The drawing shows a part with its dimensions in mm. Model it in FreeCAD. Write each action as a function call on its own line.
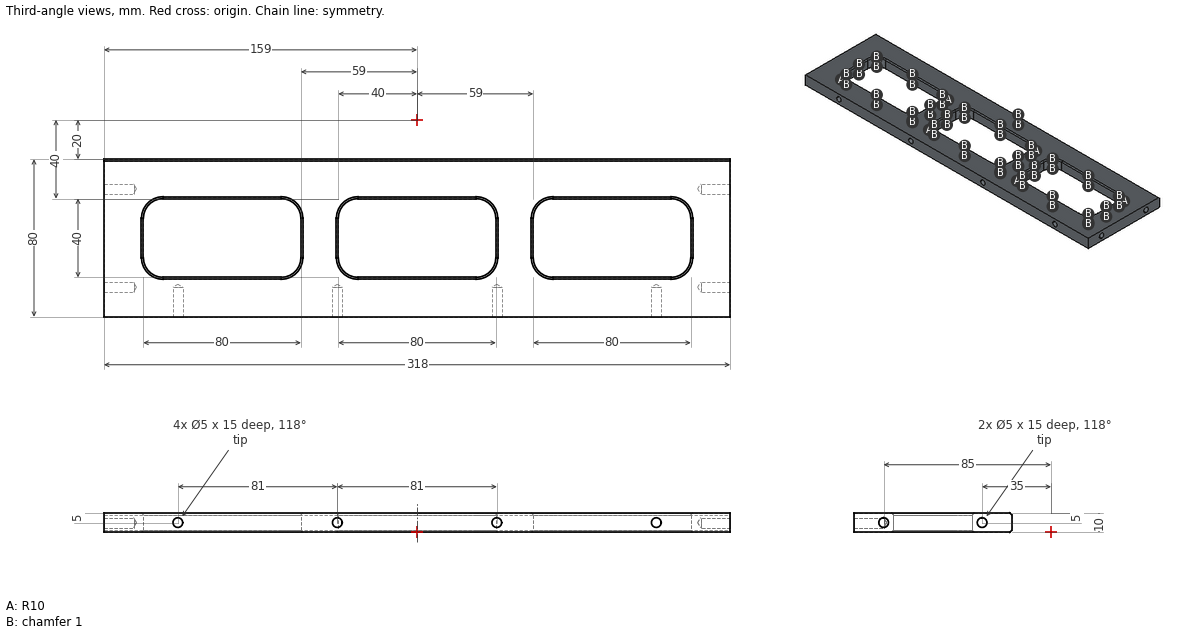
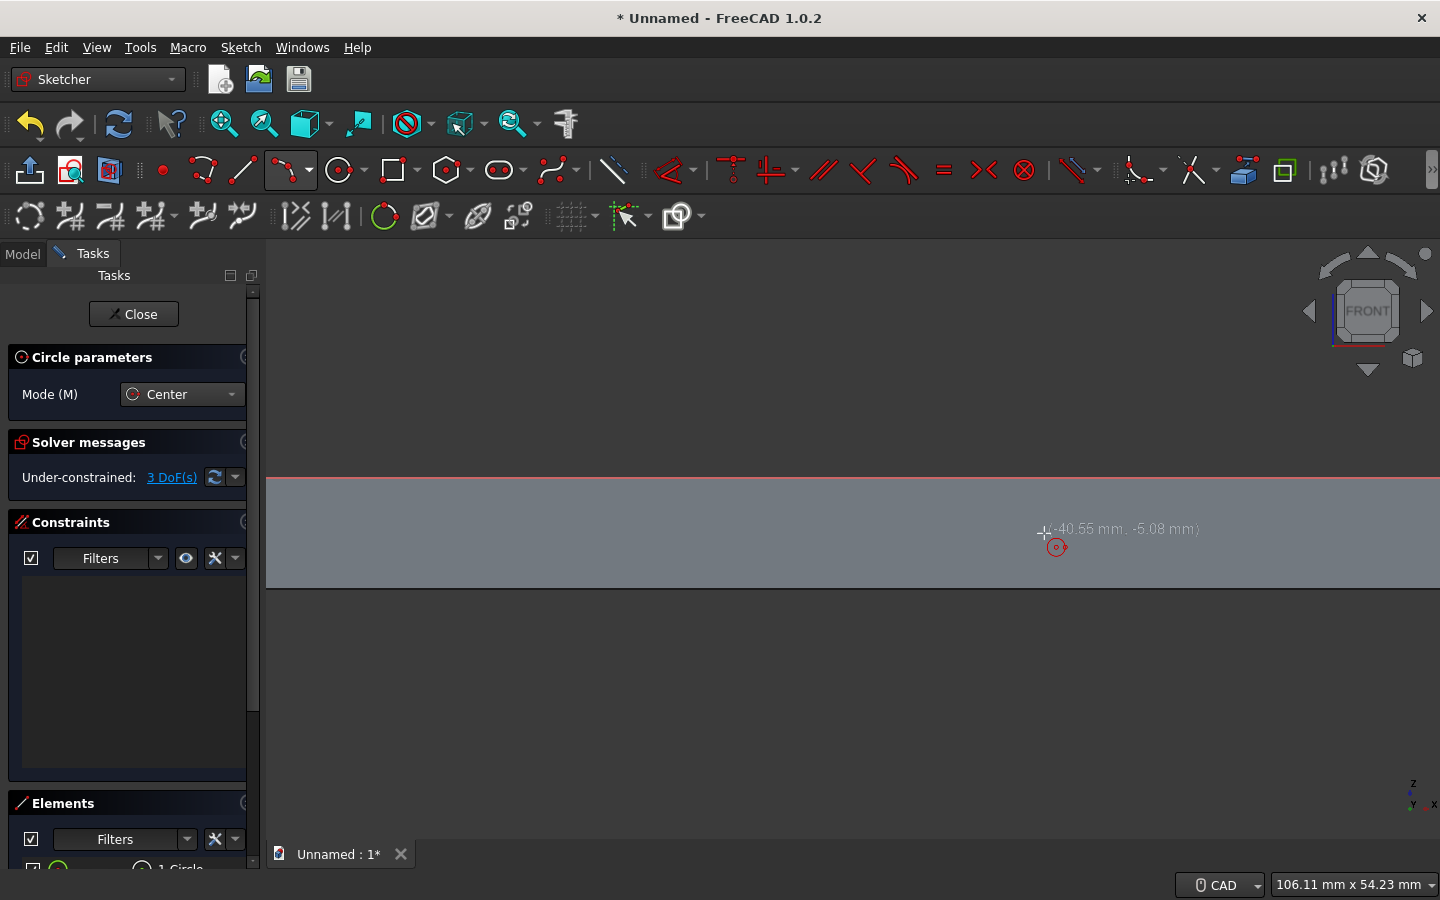
scroll(553, 545, down, 7)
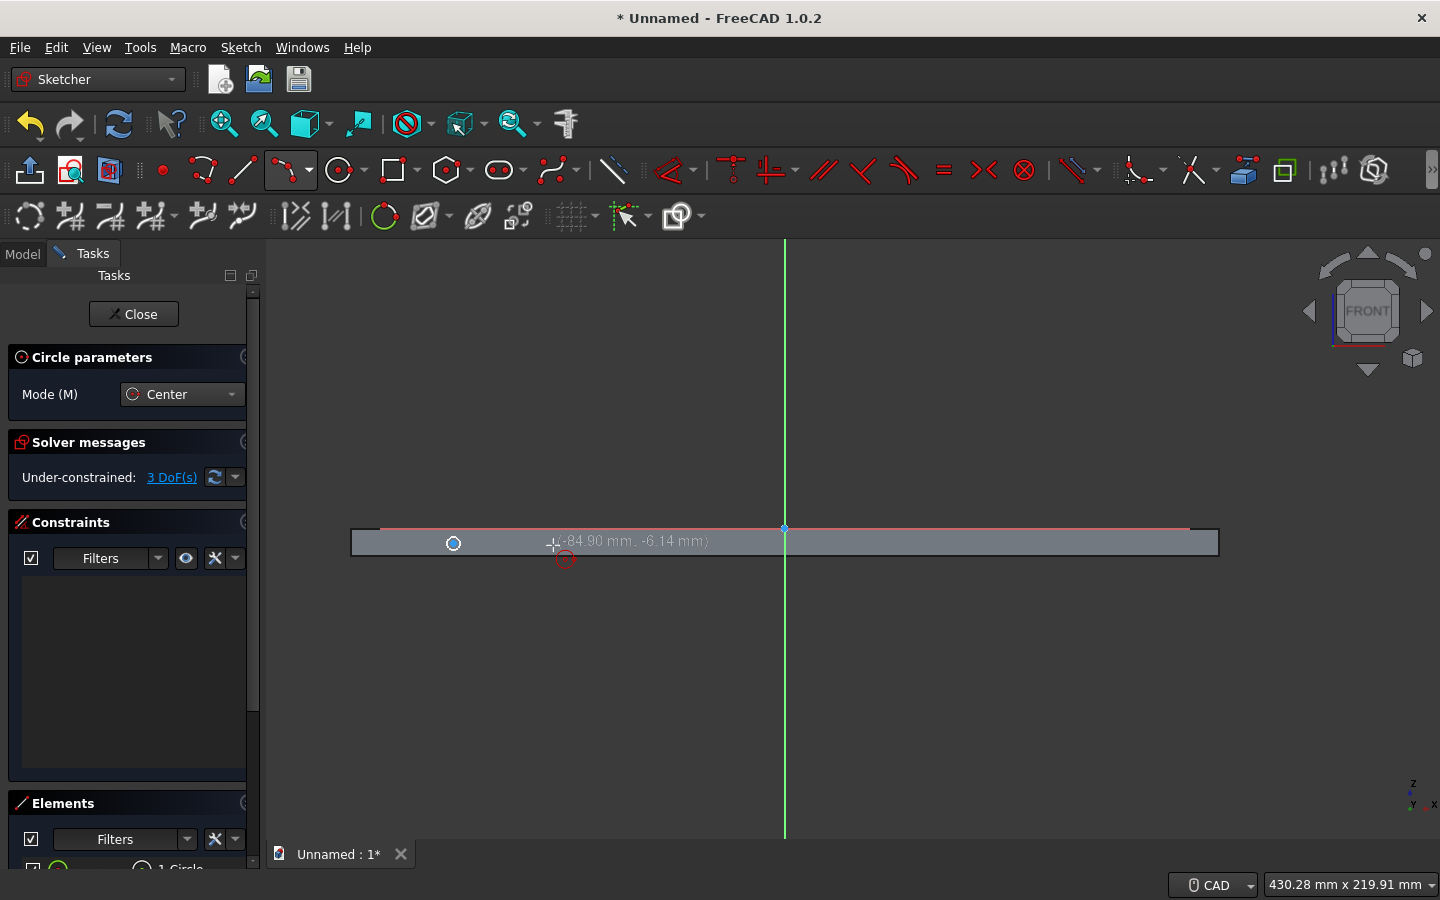
click(674, 543)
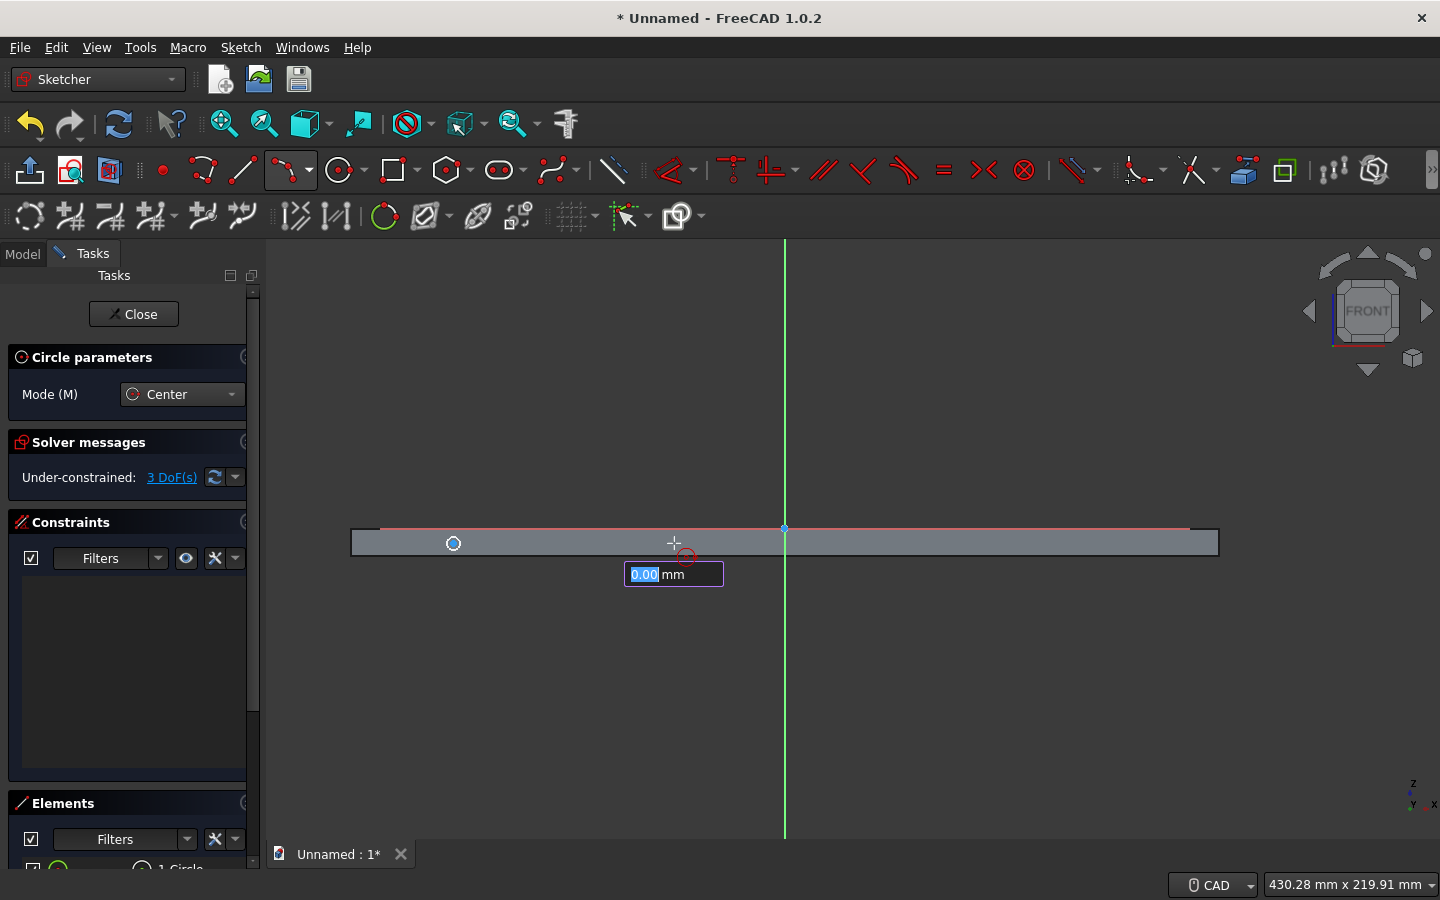
scroll(679, 547, up, 5)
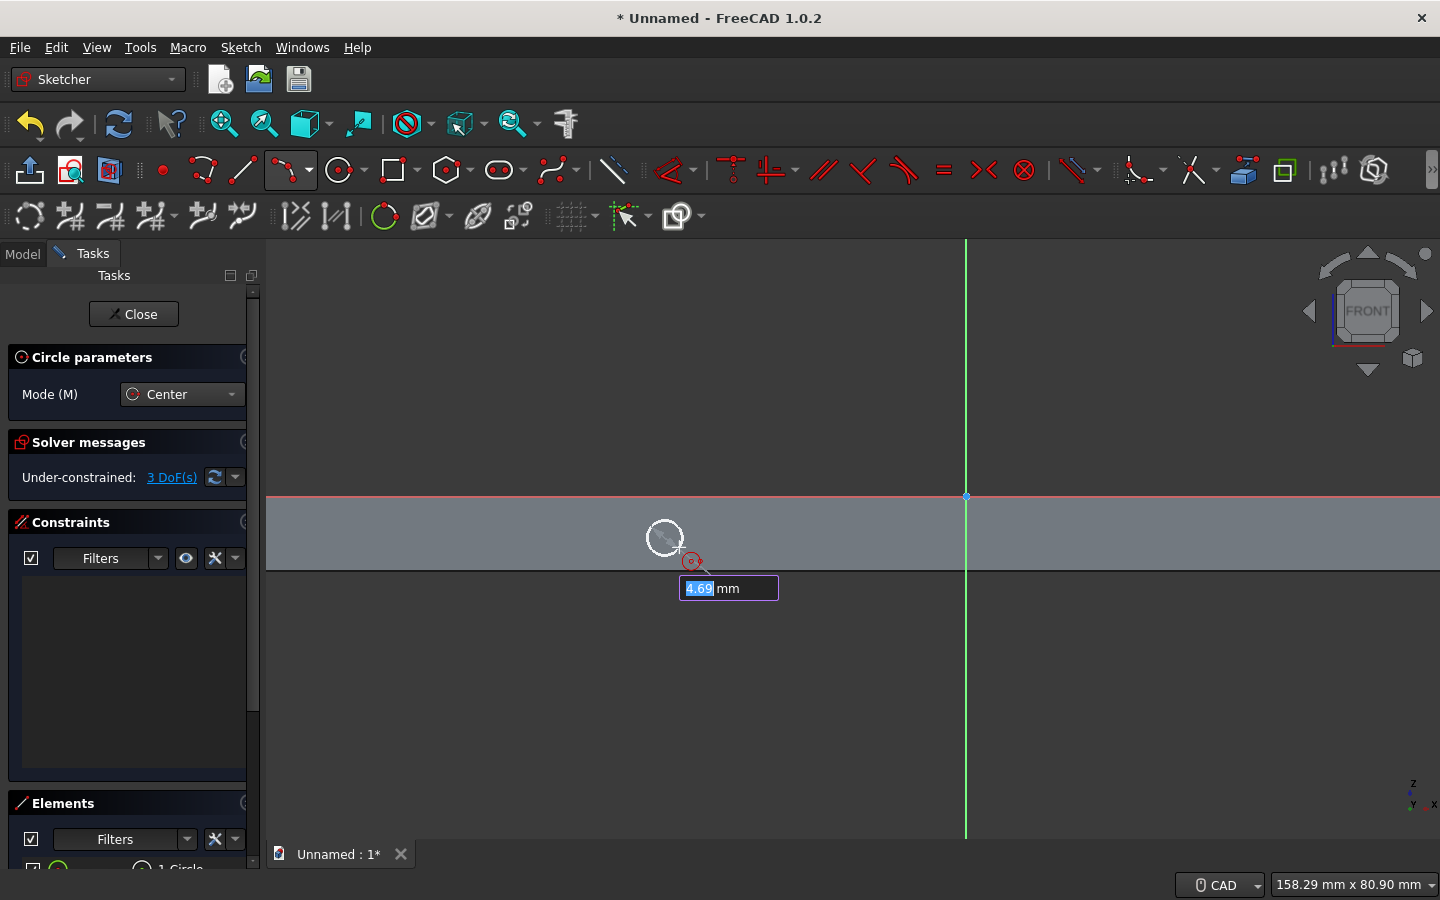
click(679, 547)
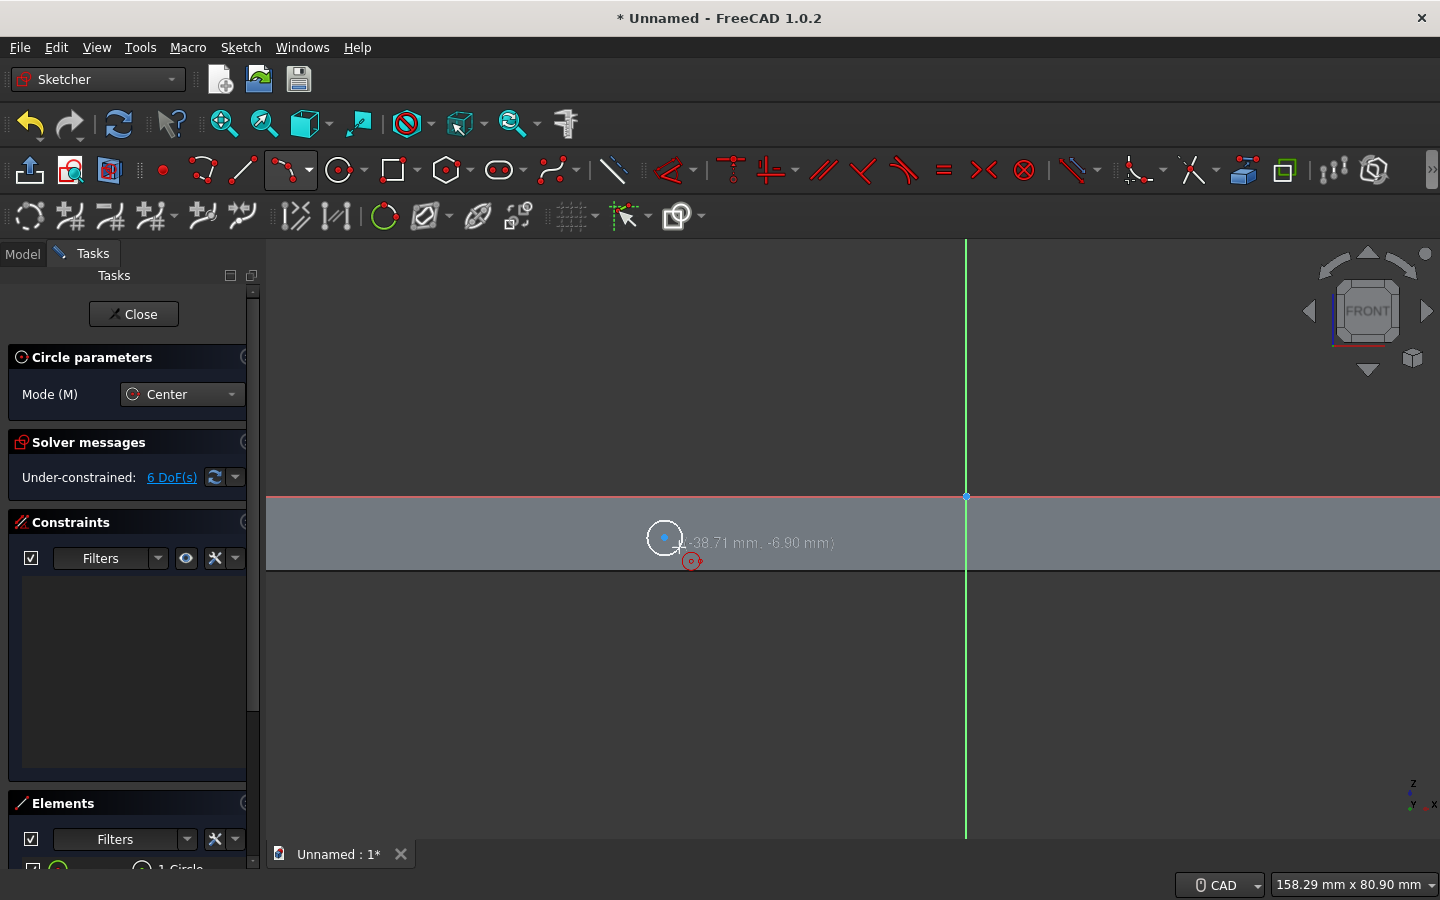
scroll(1266, 534, up, 2)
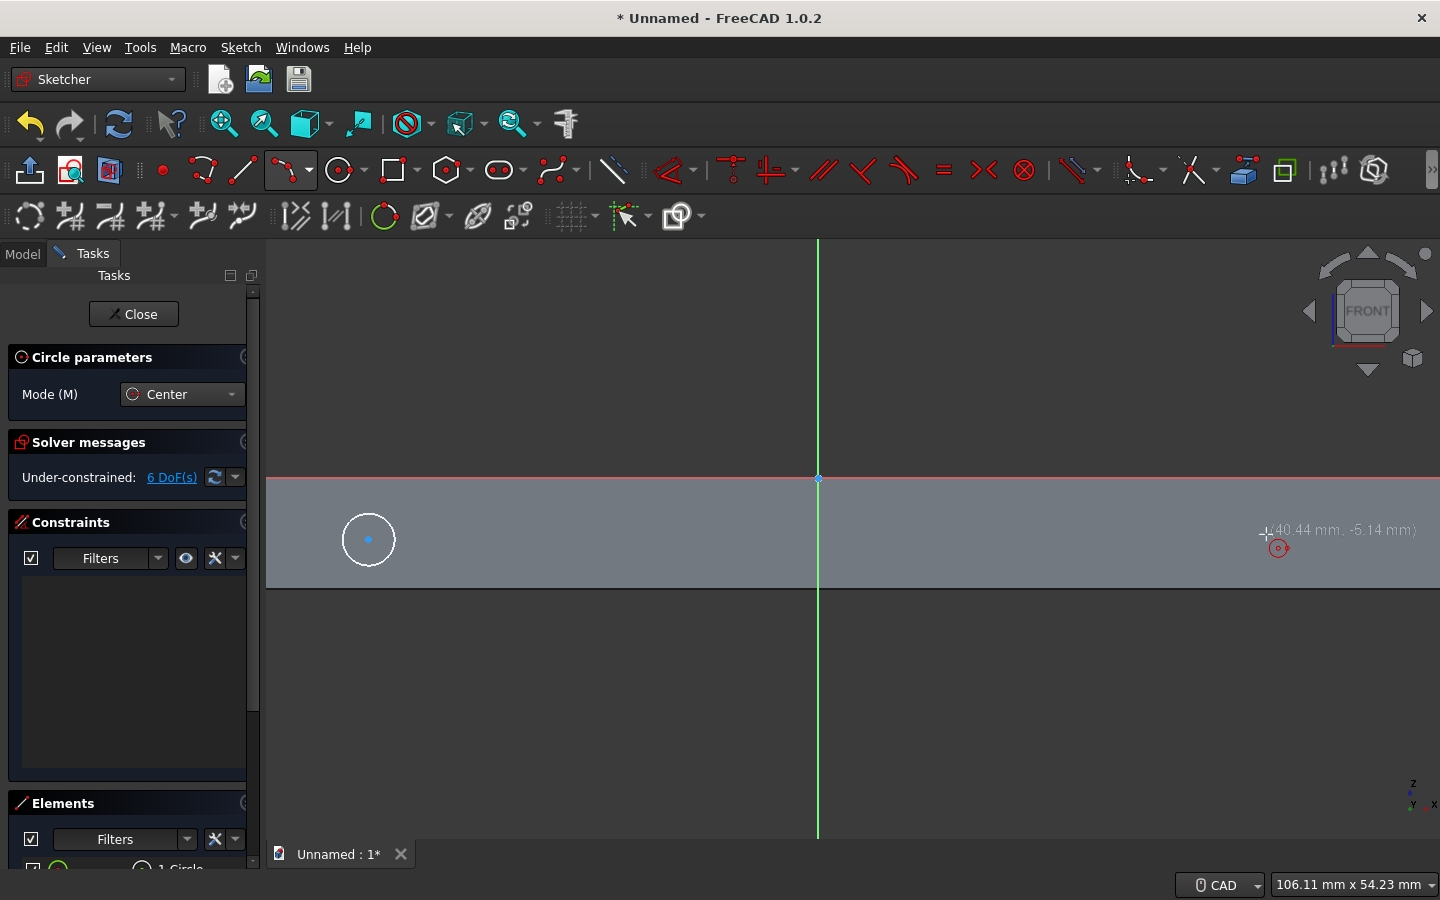
scroll(773, 545, down, 7)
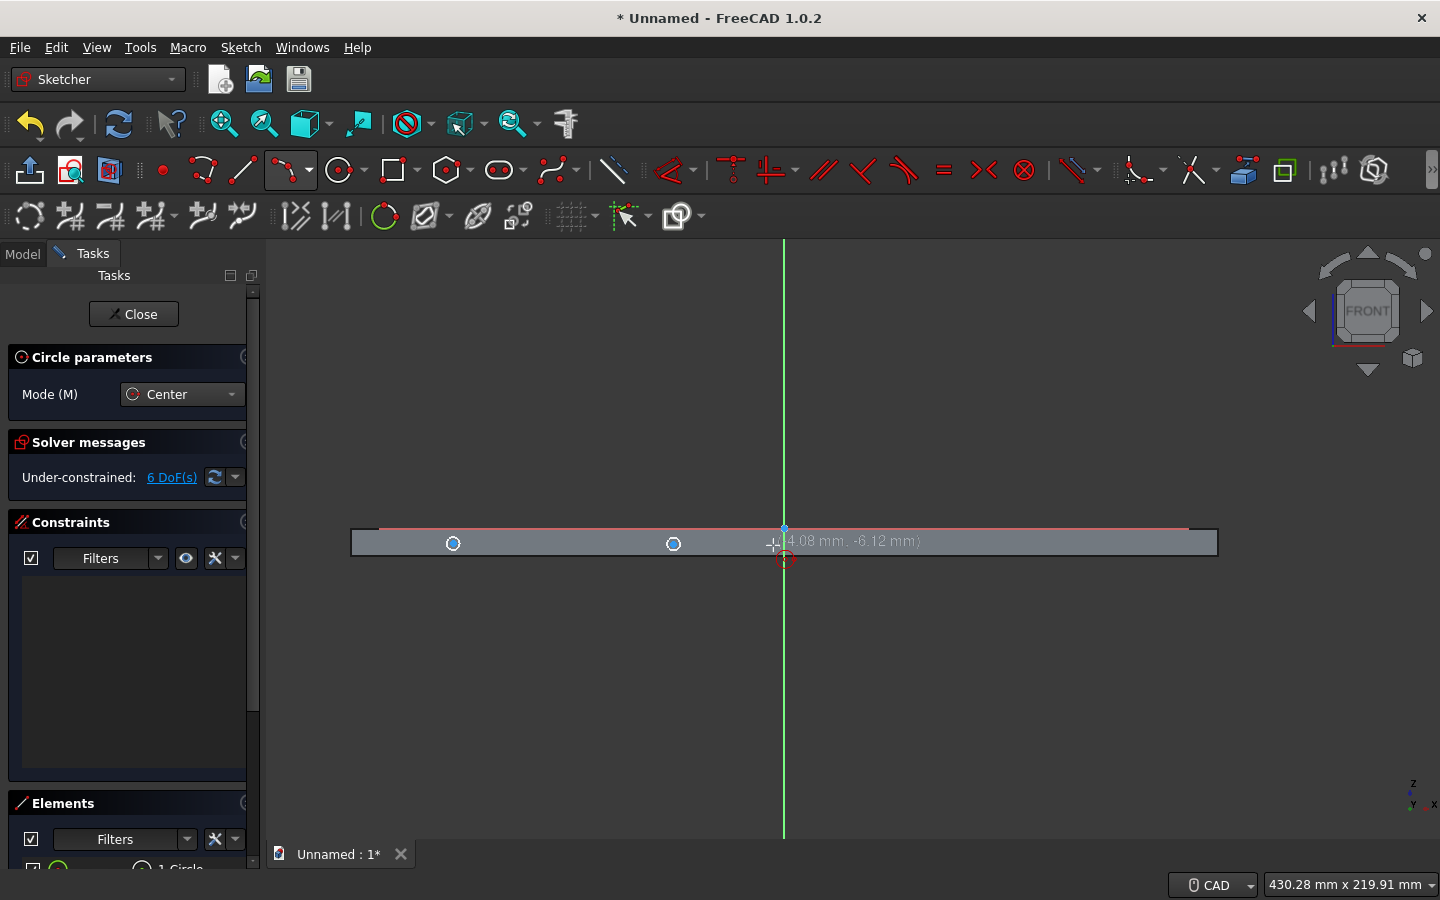
click(895, 543)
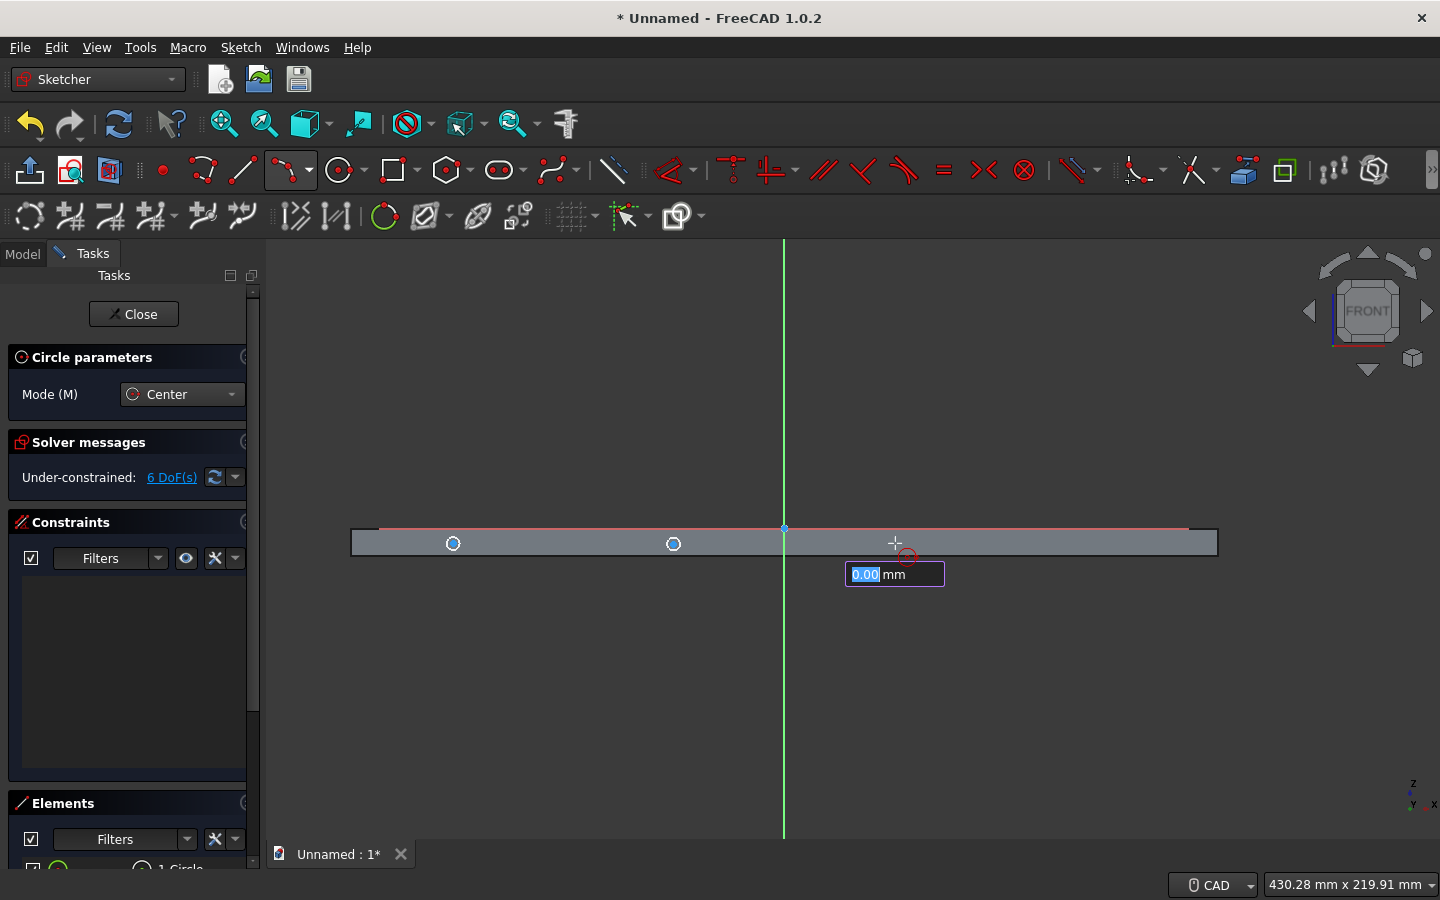
scroll(900, 547, up, 5)